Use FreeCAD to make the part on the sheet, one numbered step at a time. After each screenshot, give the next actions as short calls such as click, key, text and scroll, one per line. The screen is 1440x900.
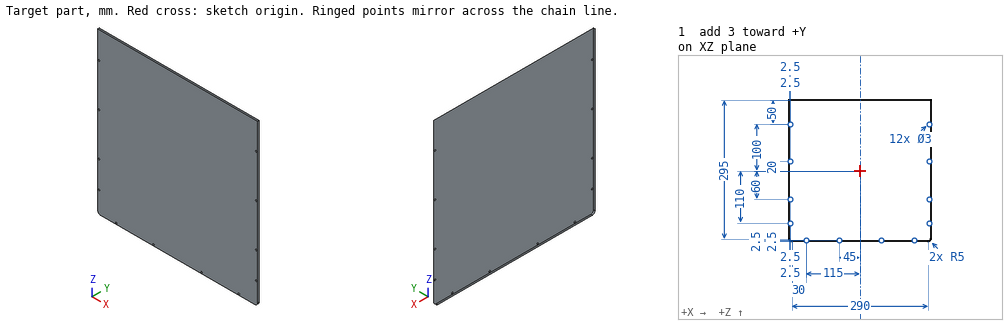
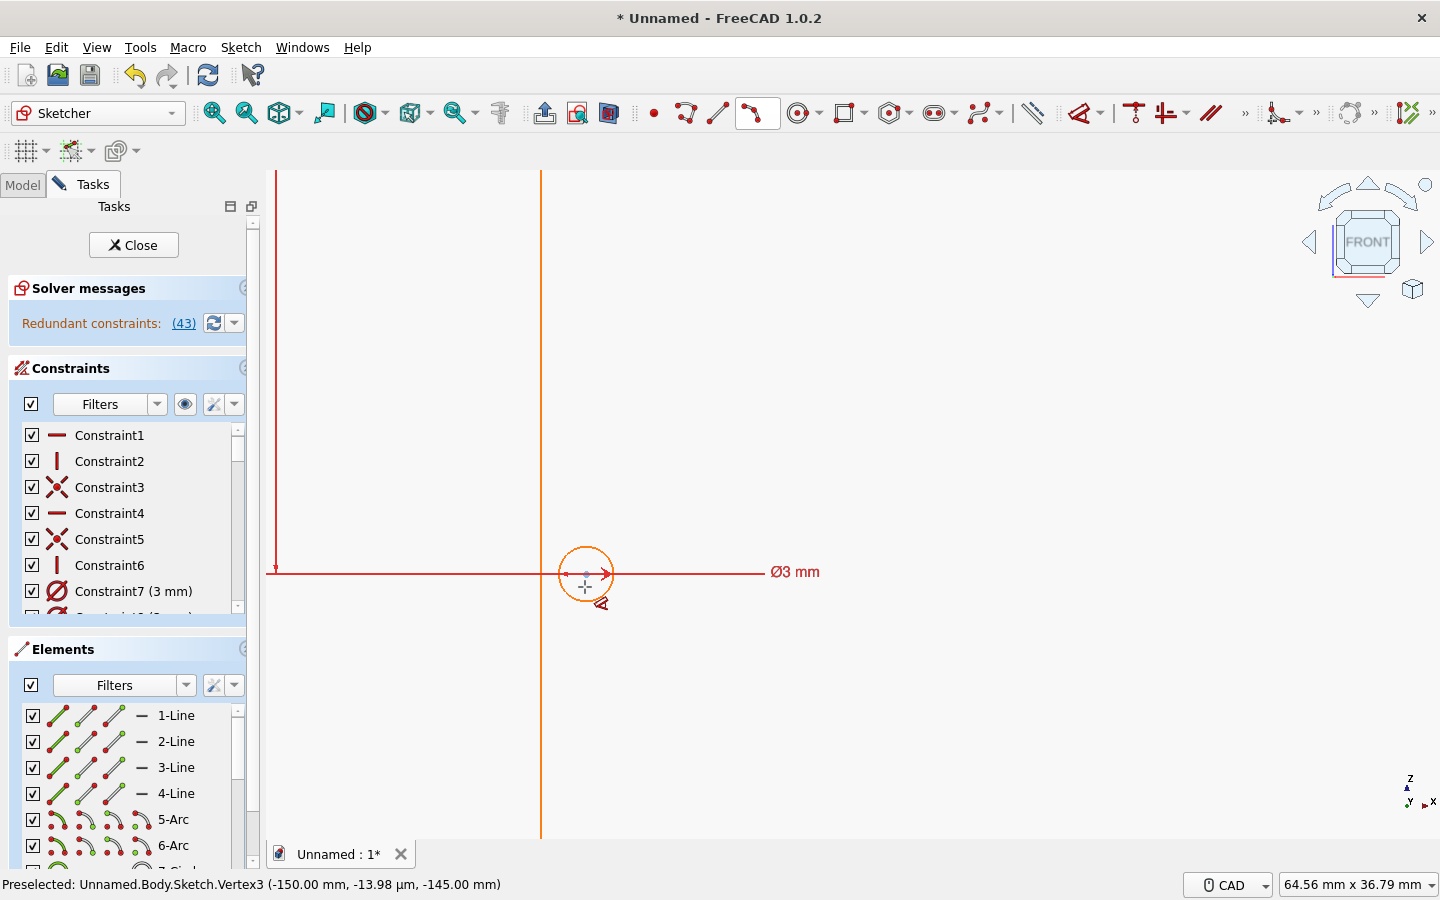
click(586, 574)
click(564, 540)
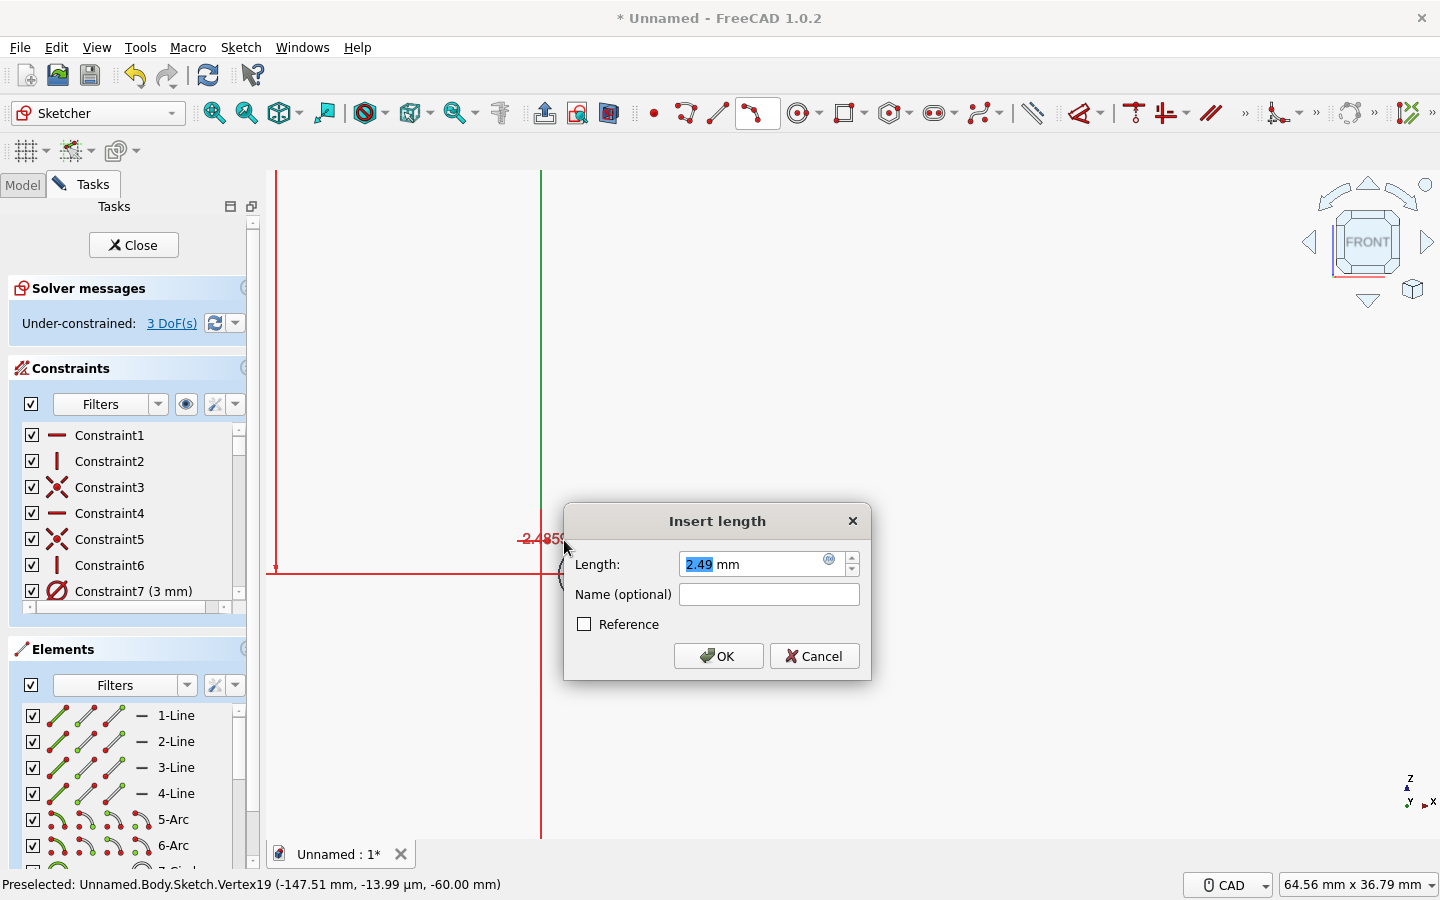
text(2.5)
key(Return)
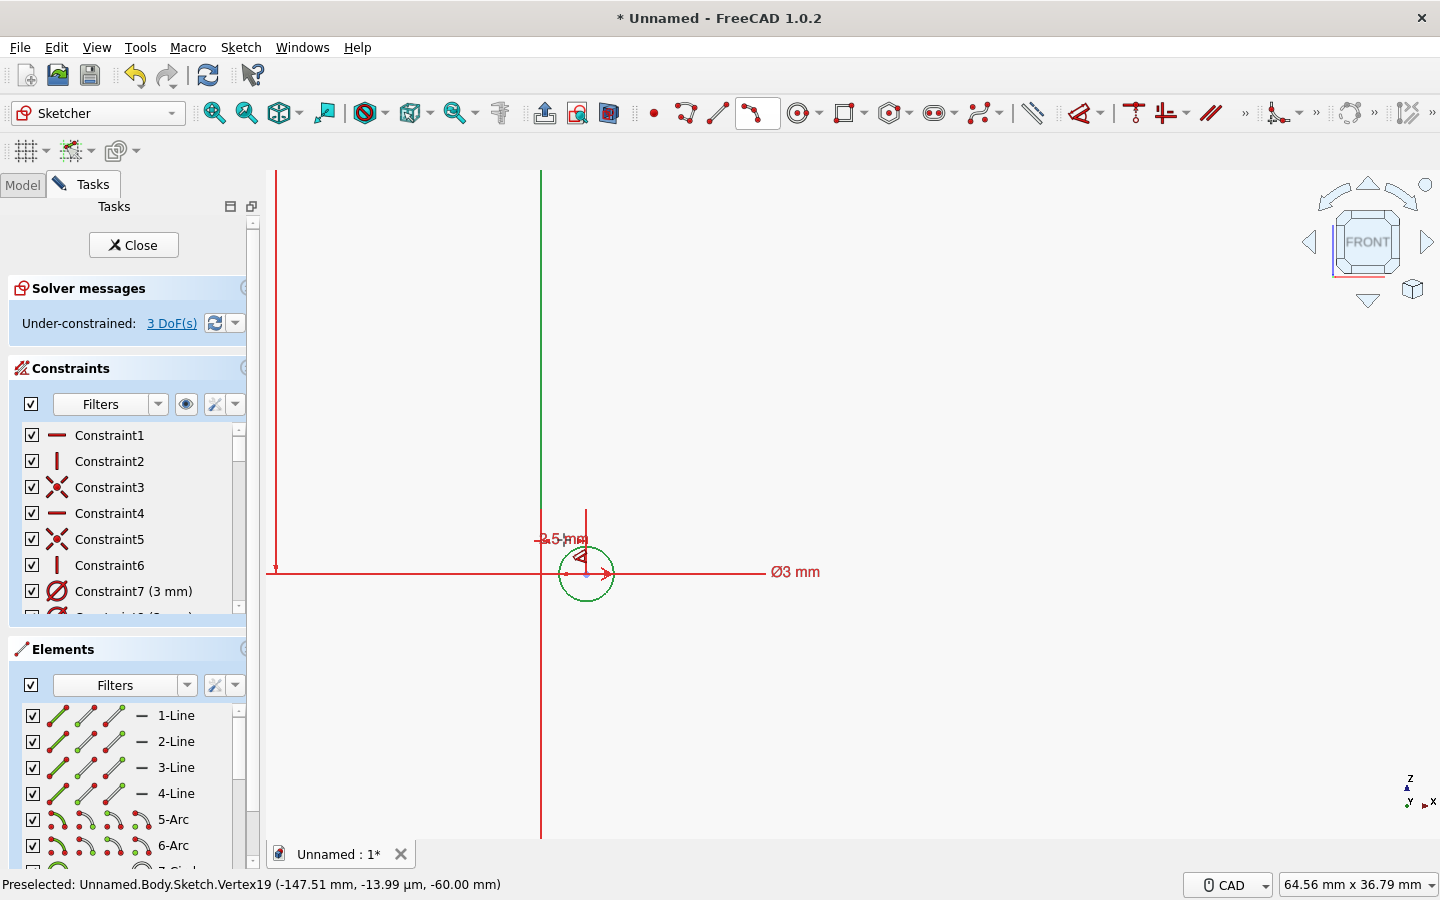
scroll(585, 586, down, 13)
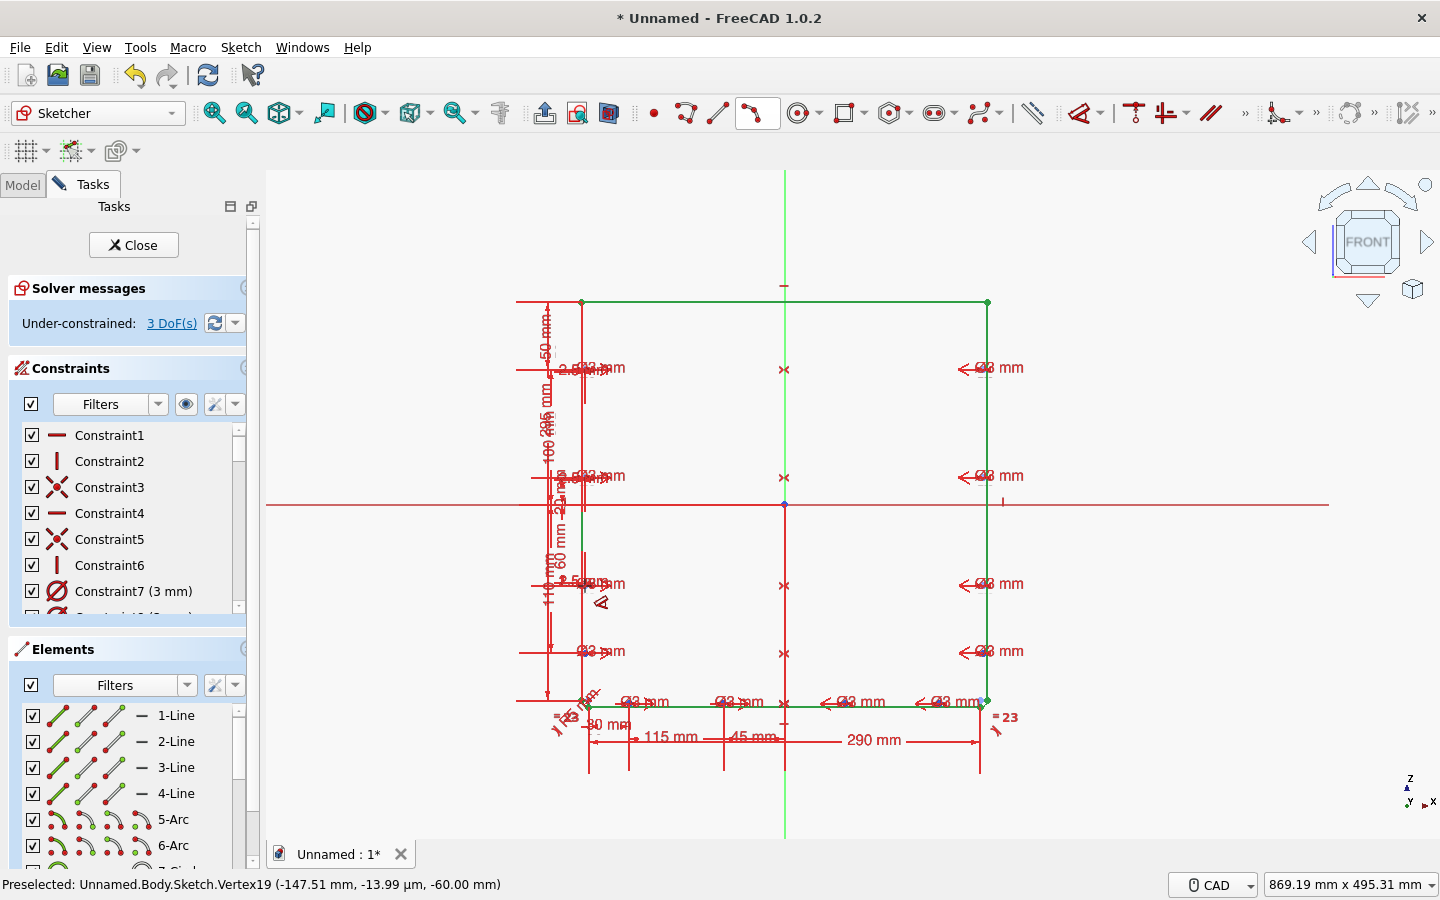
scroll(582, 700, up, 13)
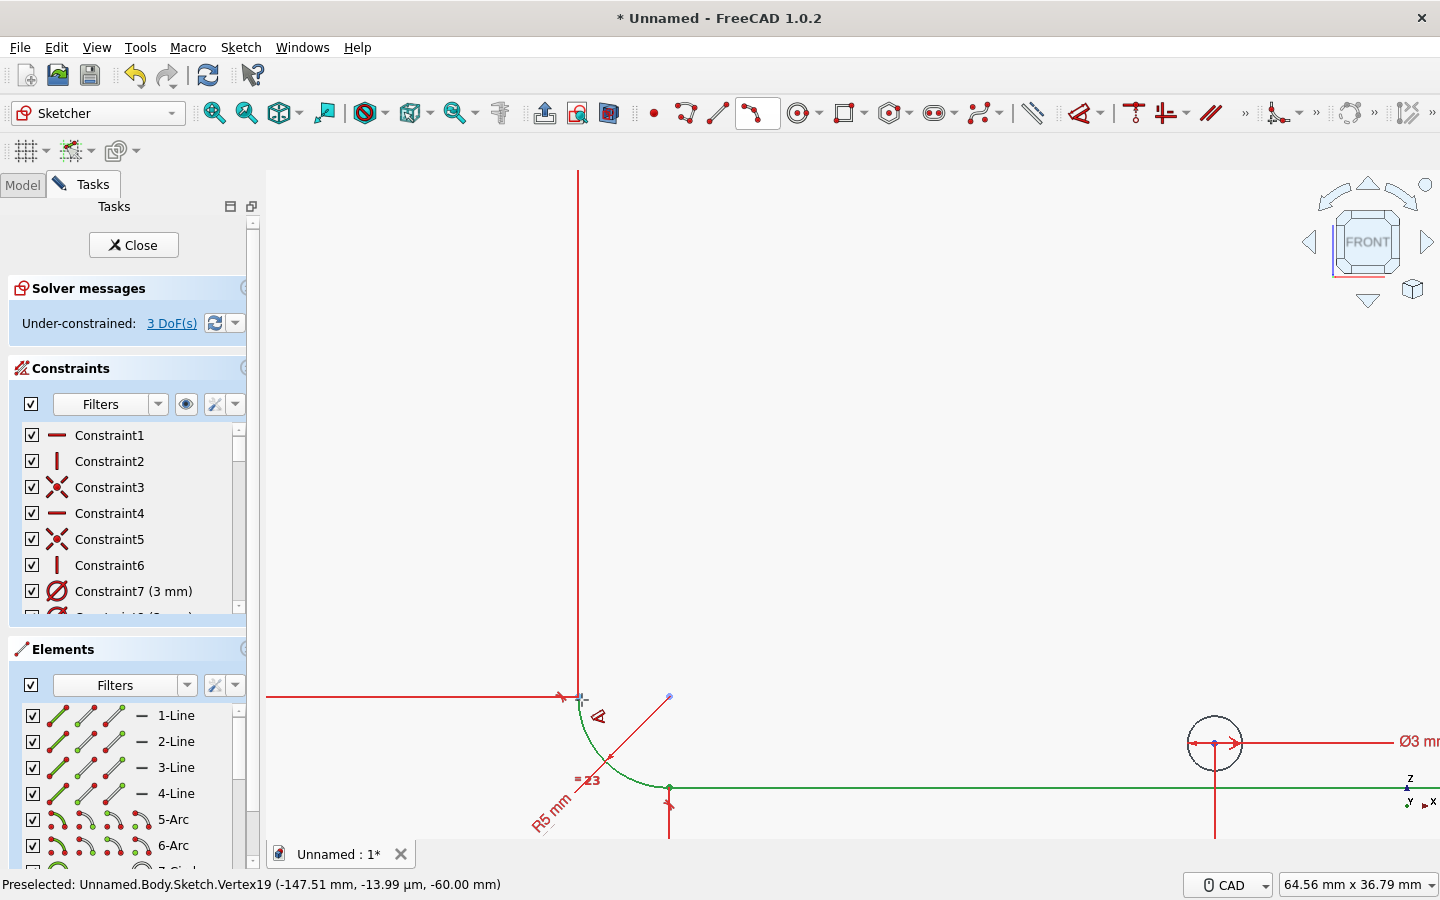
click(578, 697)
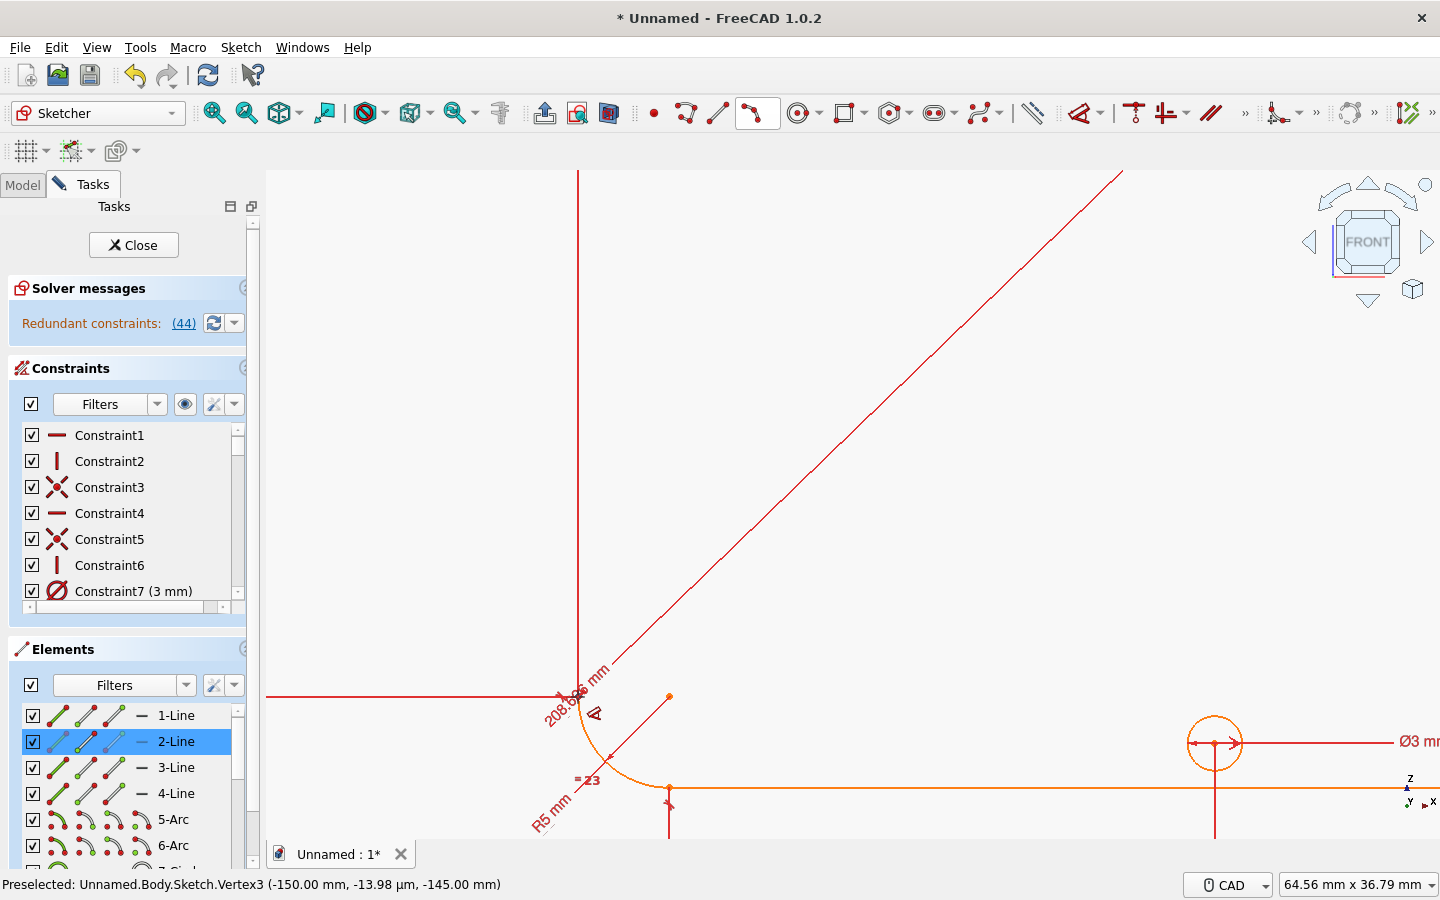
scroll(582, 701, down, 13)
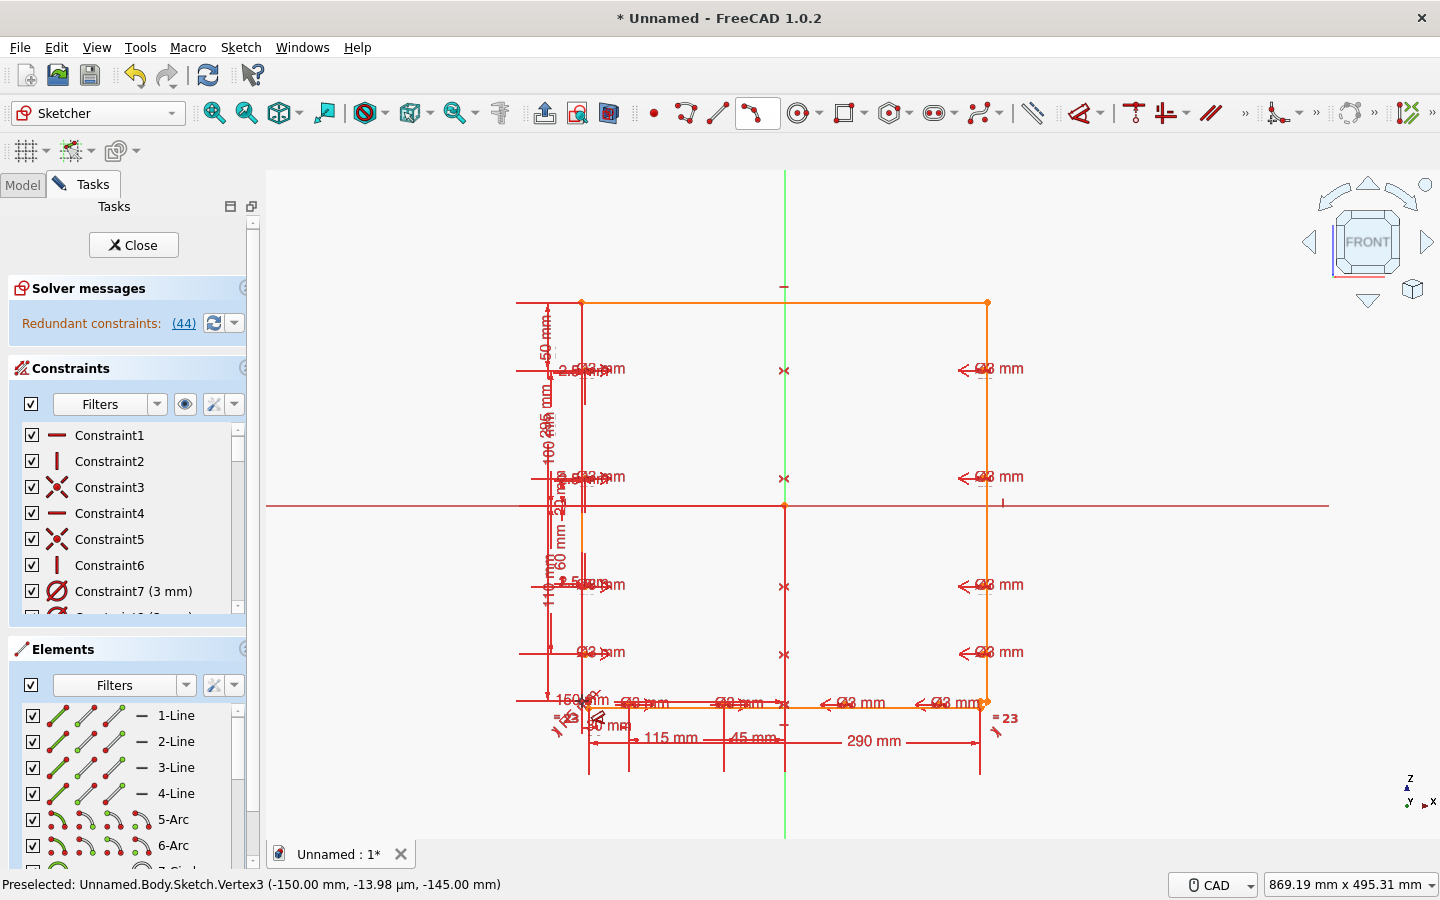
scroll(585, 654, up, 13)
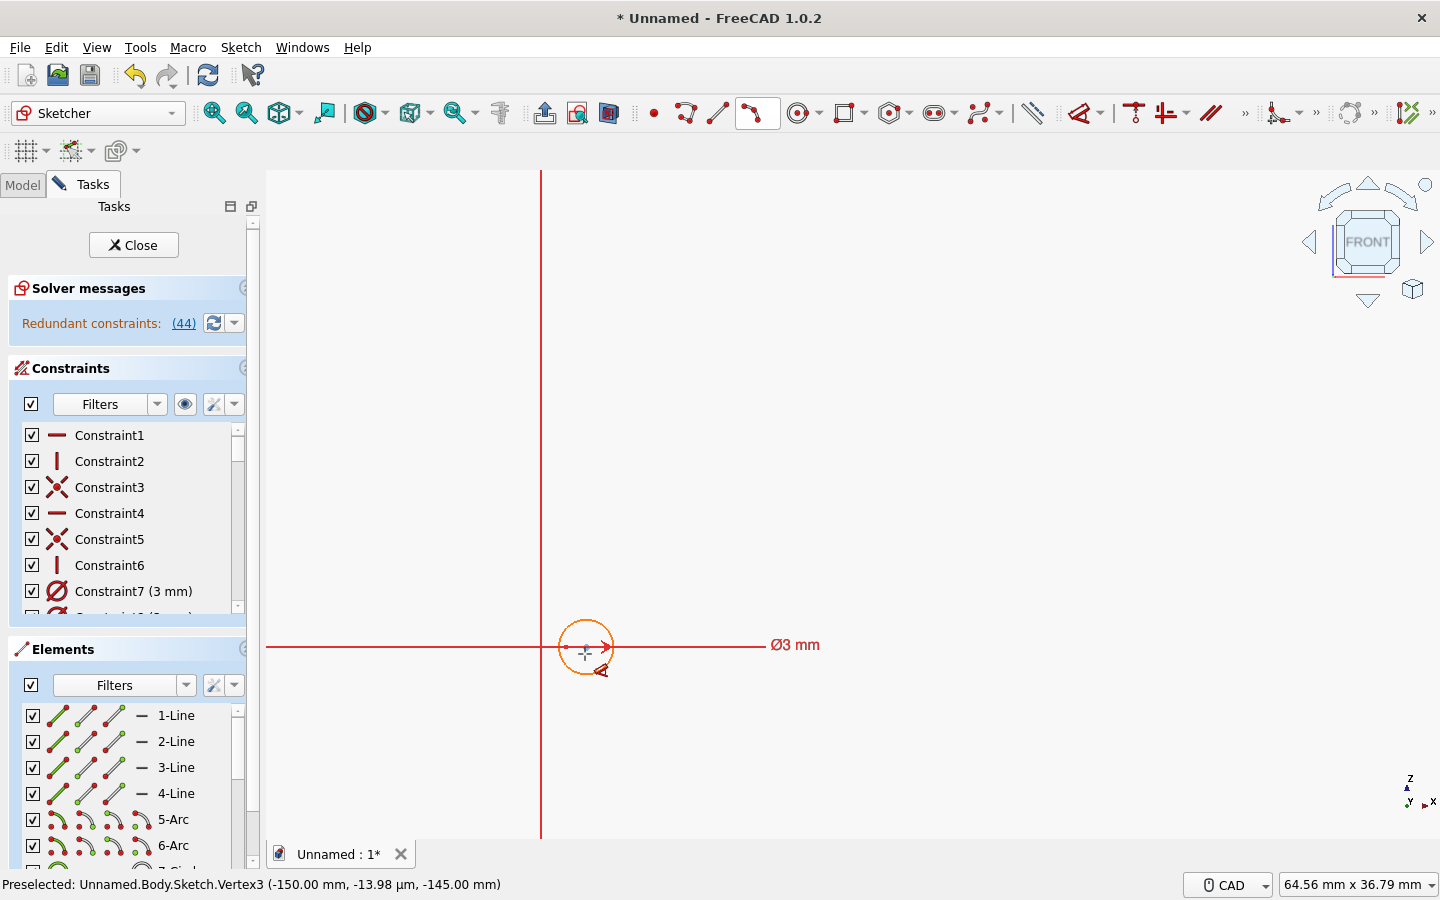
click(586, 647)
click(564, 613)